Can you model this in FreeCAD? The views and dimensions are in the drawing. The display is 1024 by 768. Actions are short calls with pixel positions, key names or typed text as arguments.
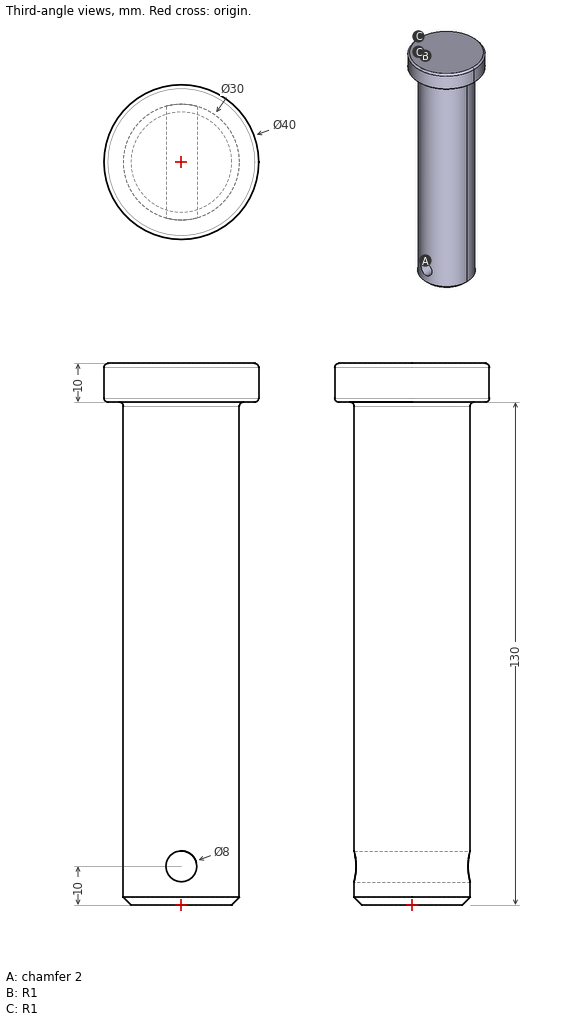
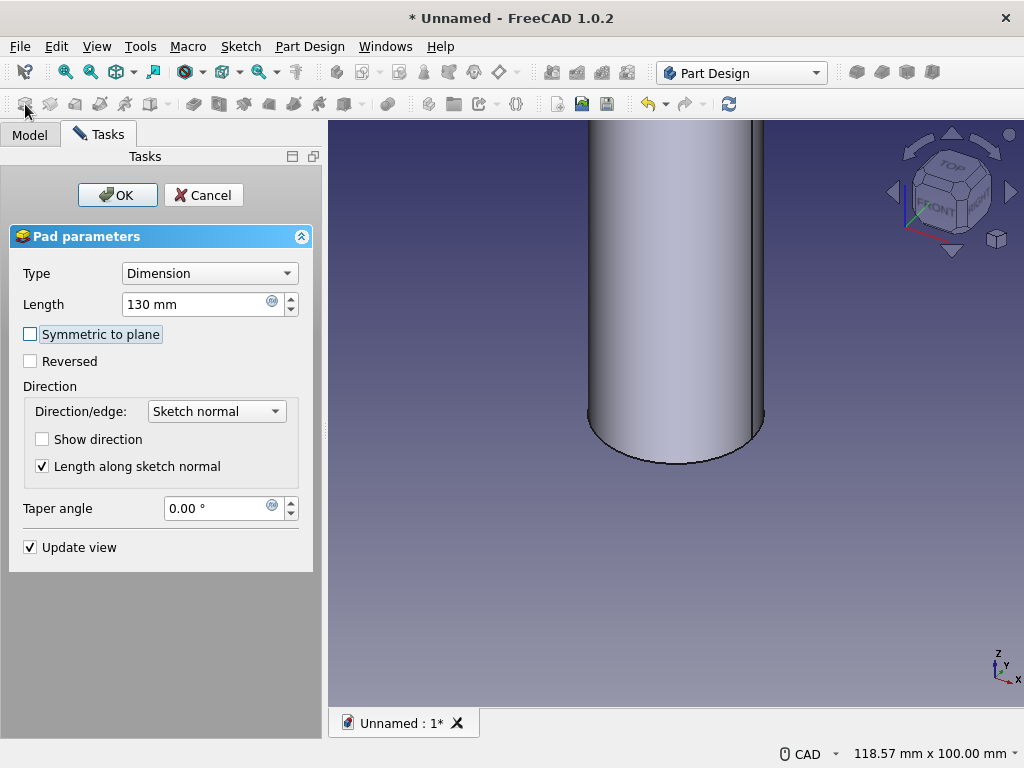
click(118, 195)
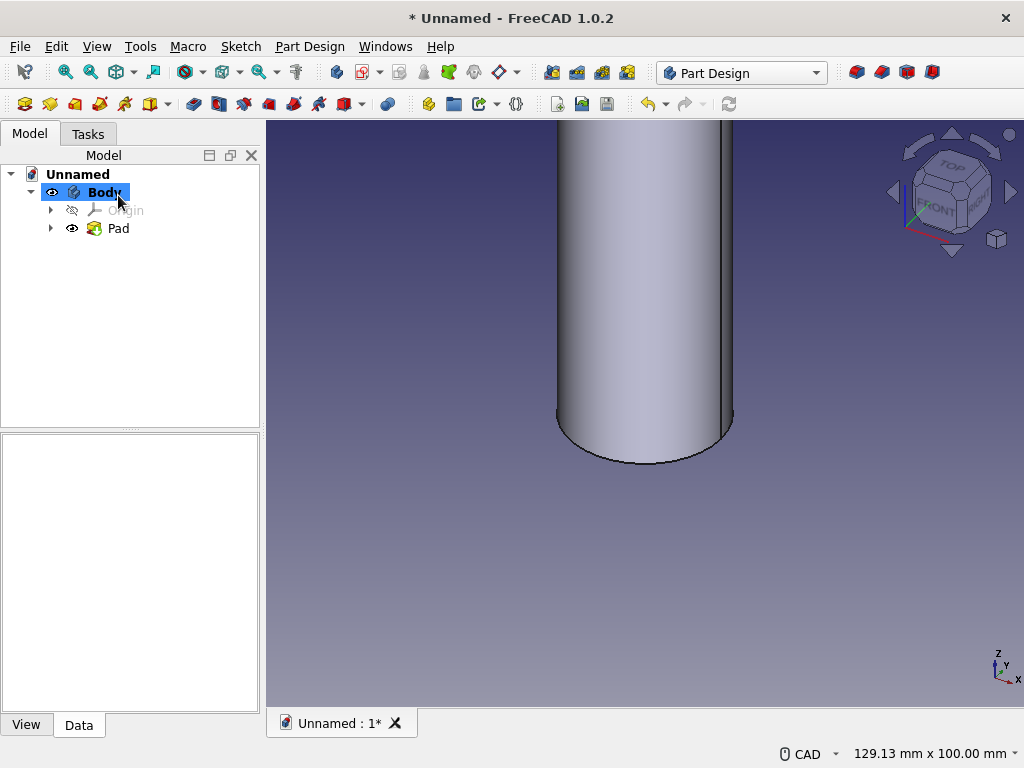
click(66, 72)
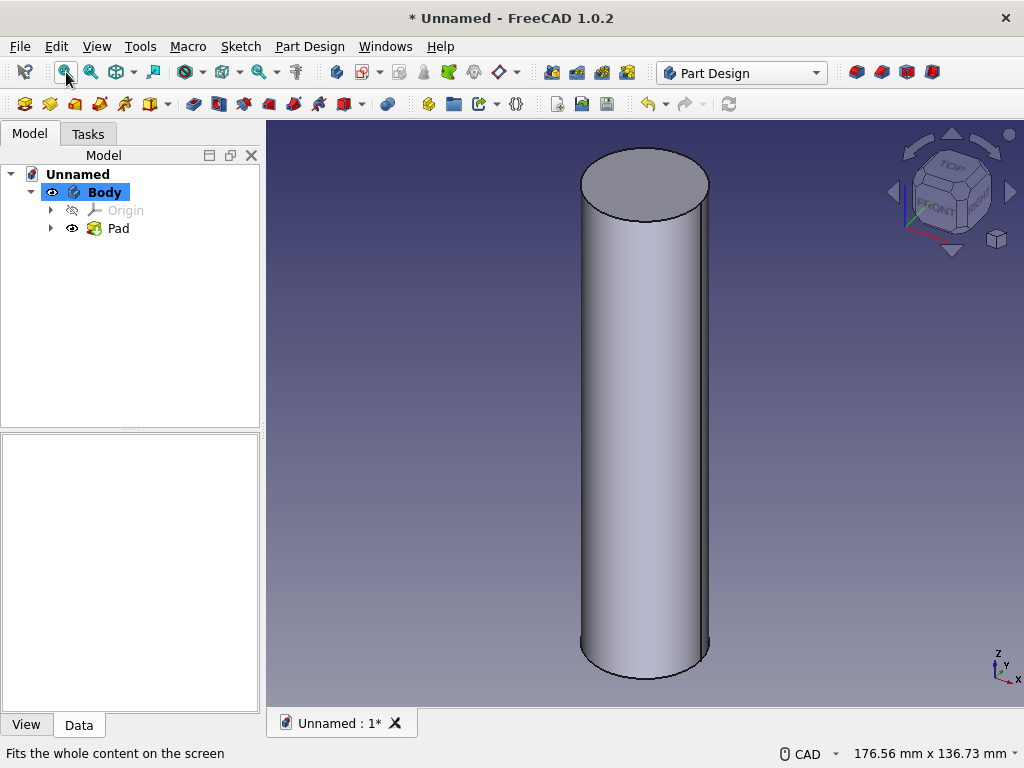
click(645, 184)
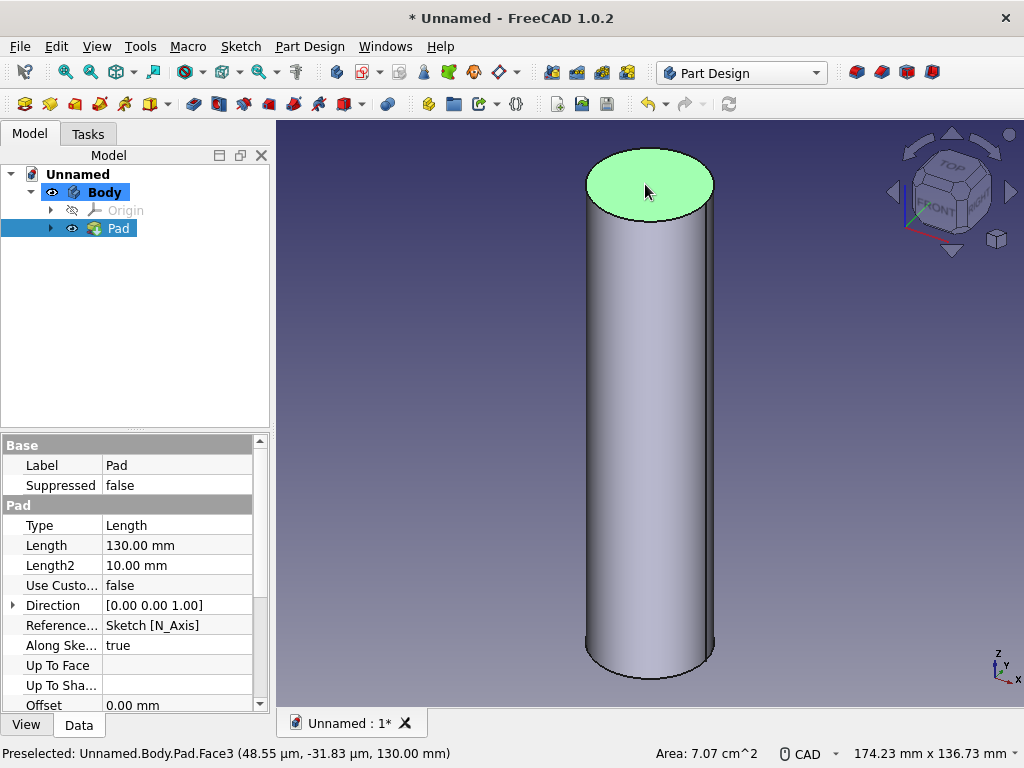
click(362, 72)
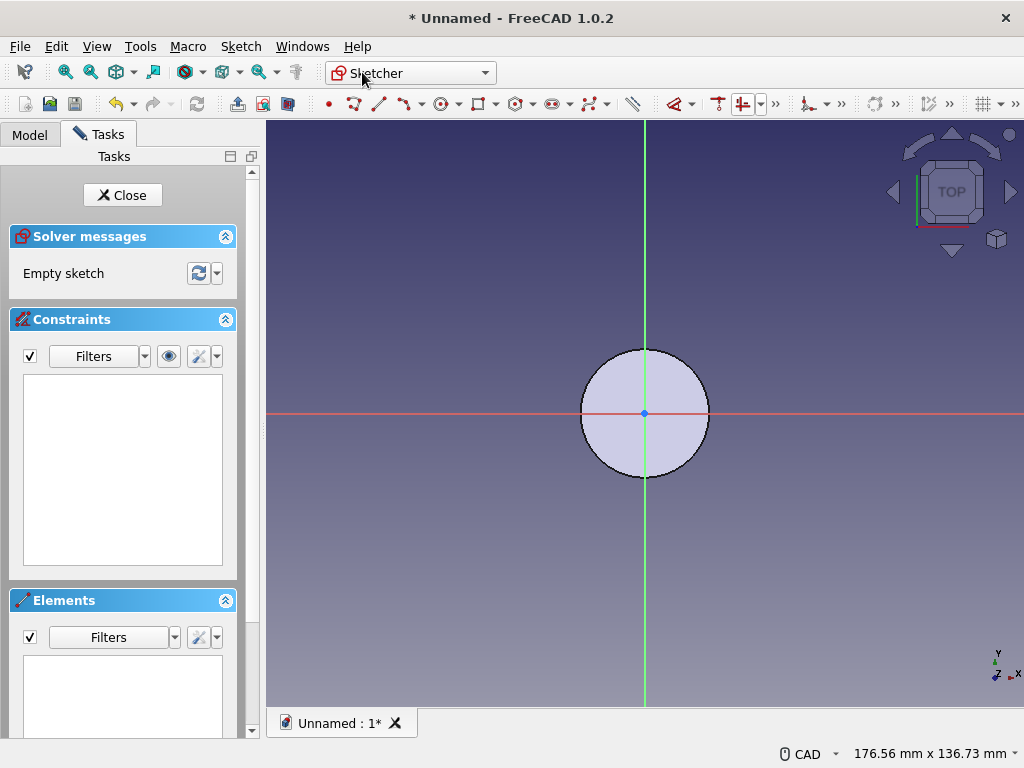
scroll(701, 413, up, 4)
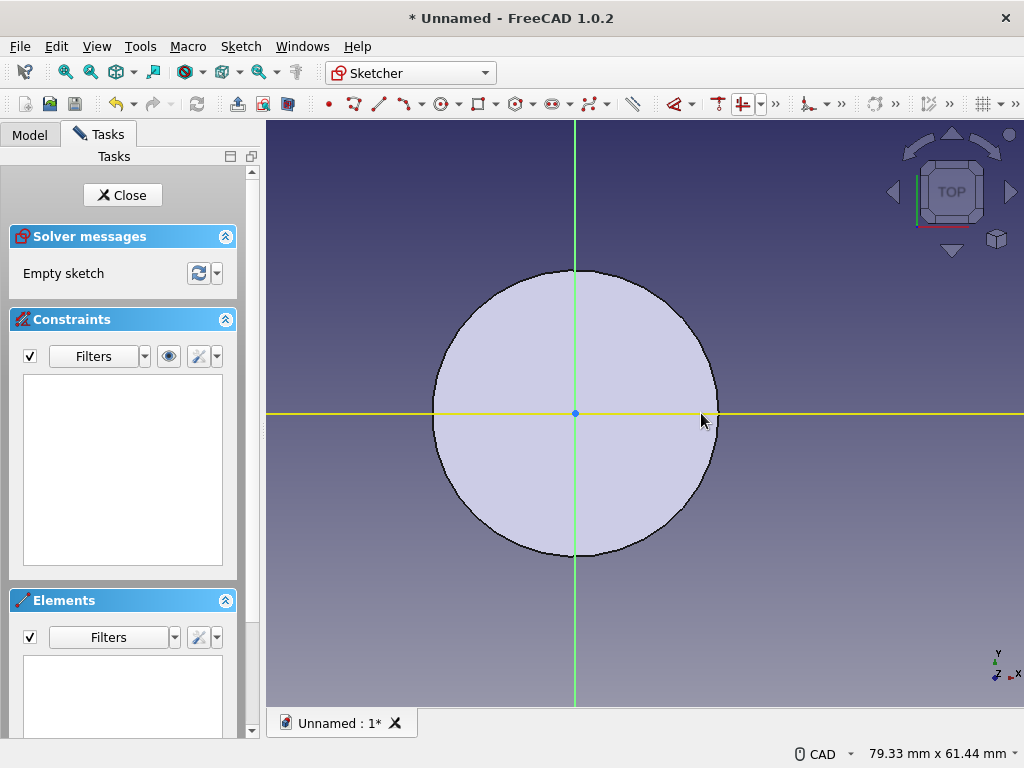
click(440, 104)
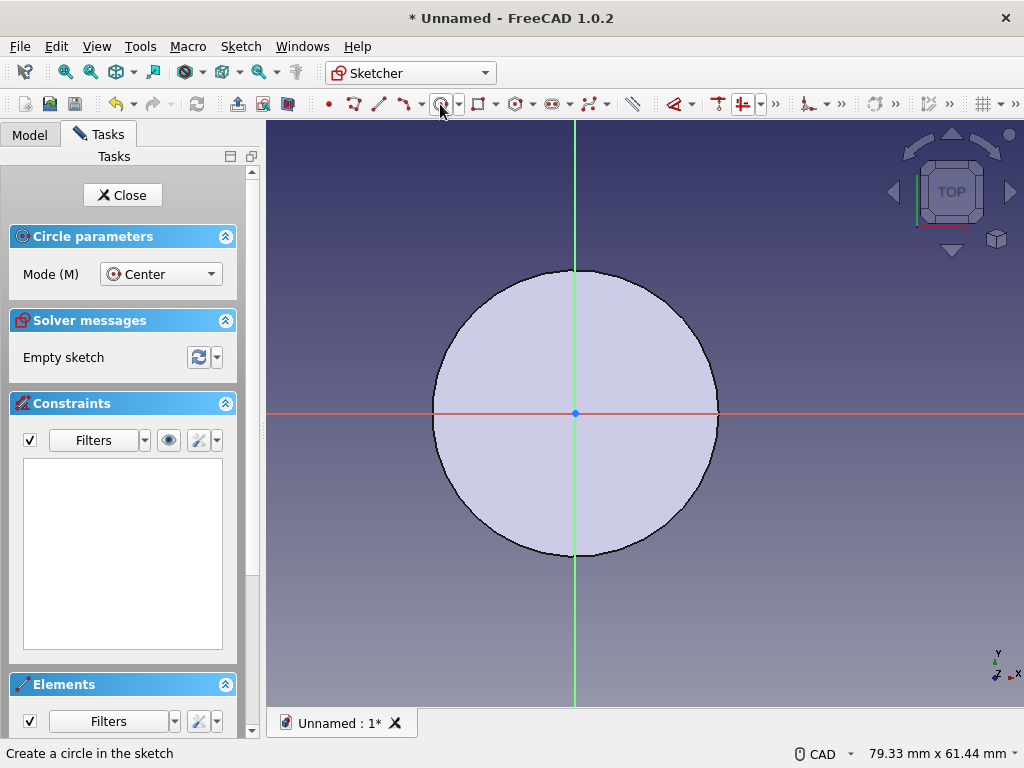
click(575, 414)
click(711, 278)
key(Escape)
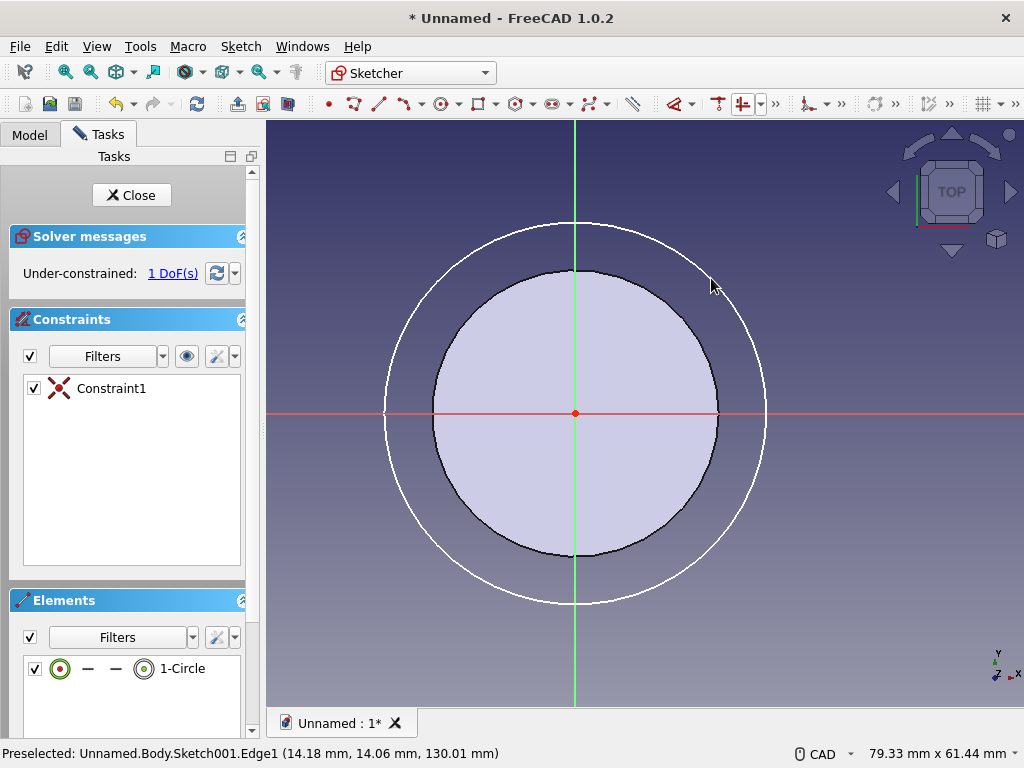
click(674, 104)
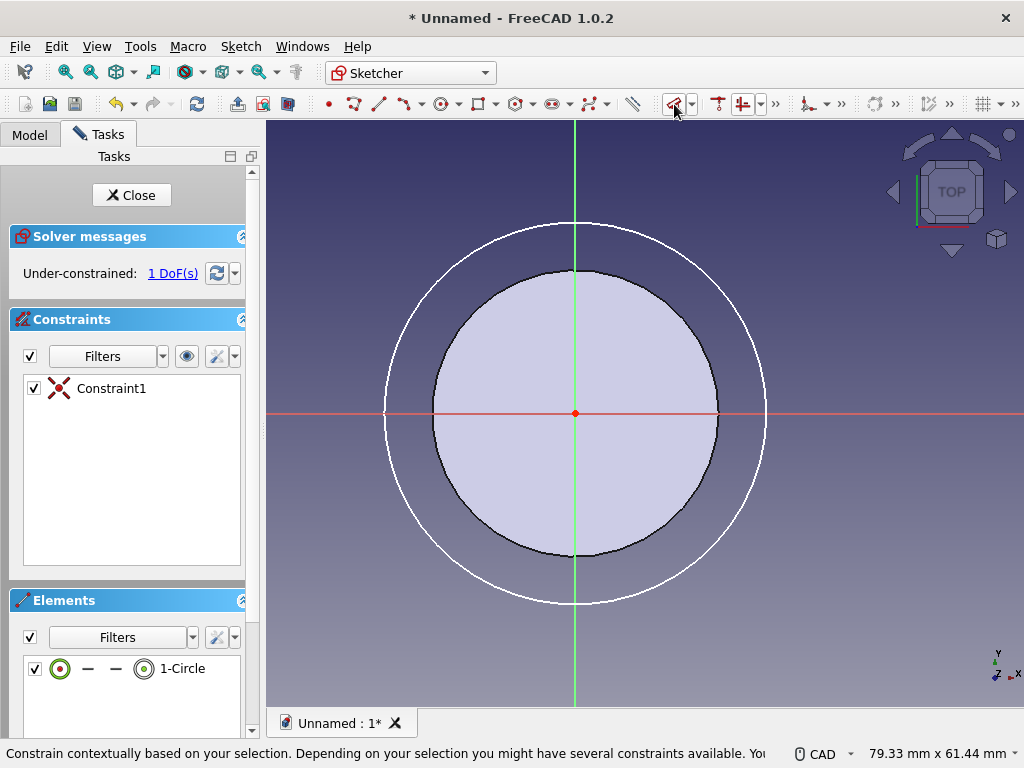
click(710, 278)
click(733, 255)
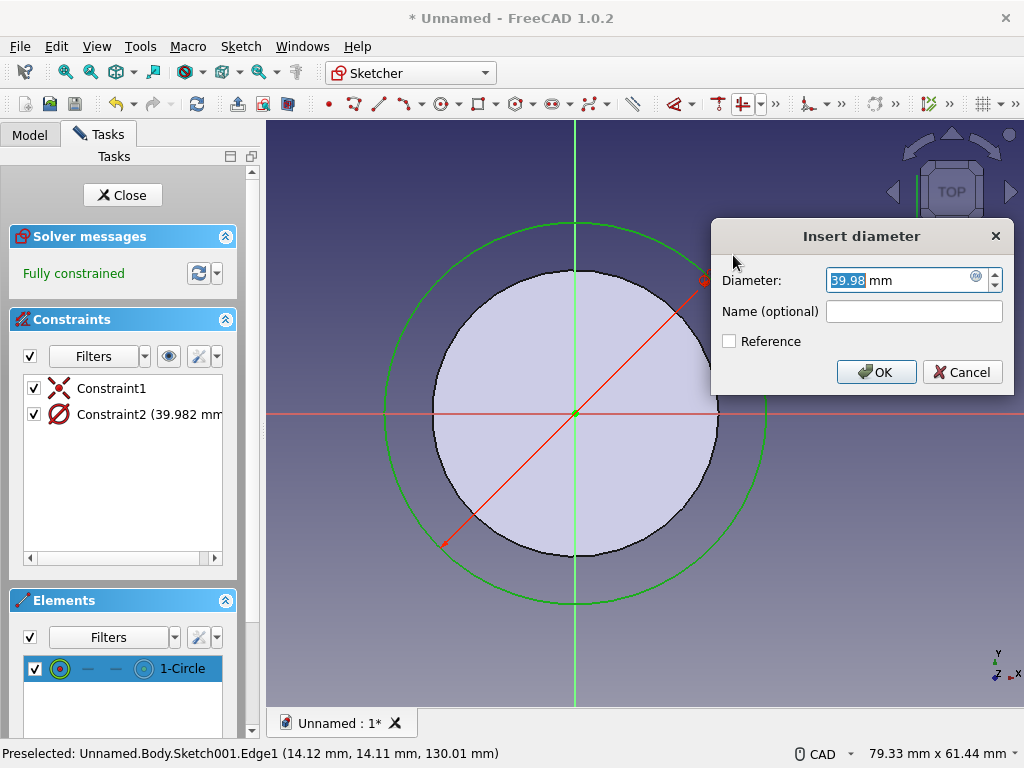
text(40)
key(Return)
key(Escape)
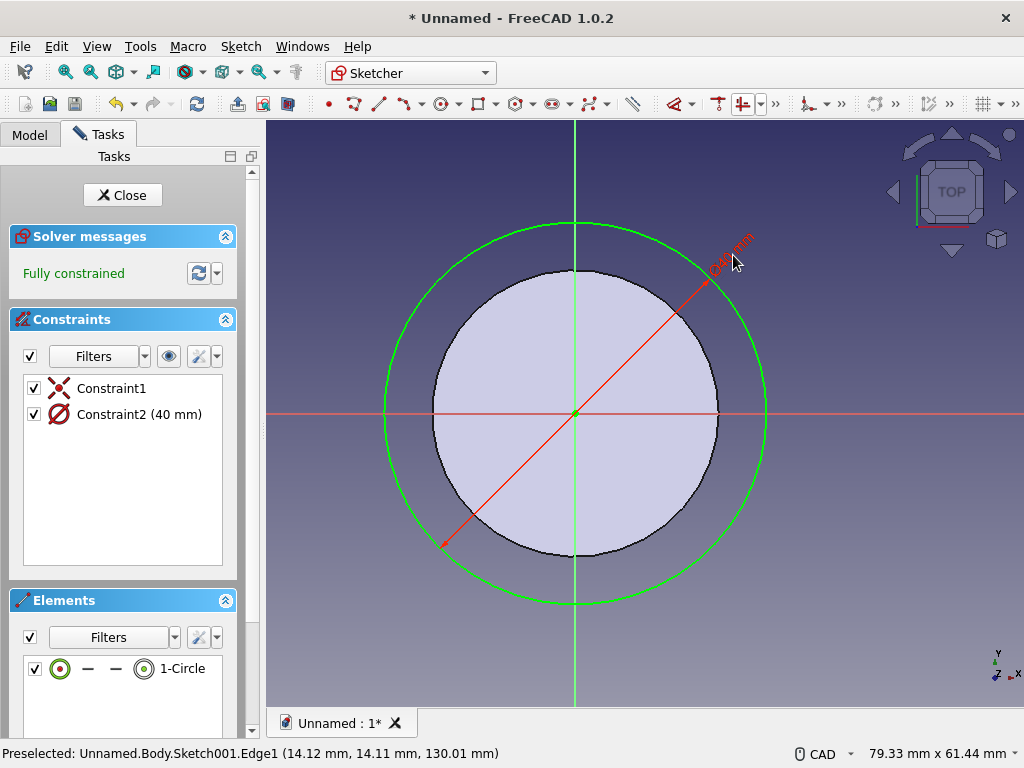
click(123, 195)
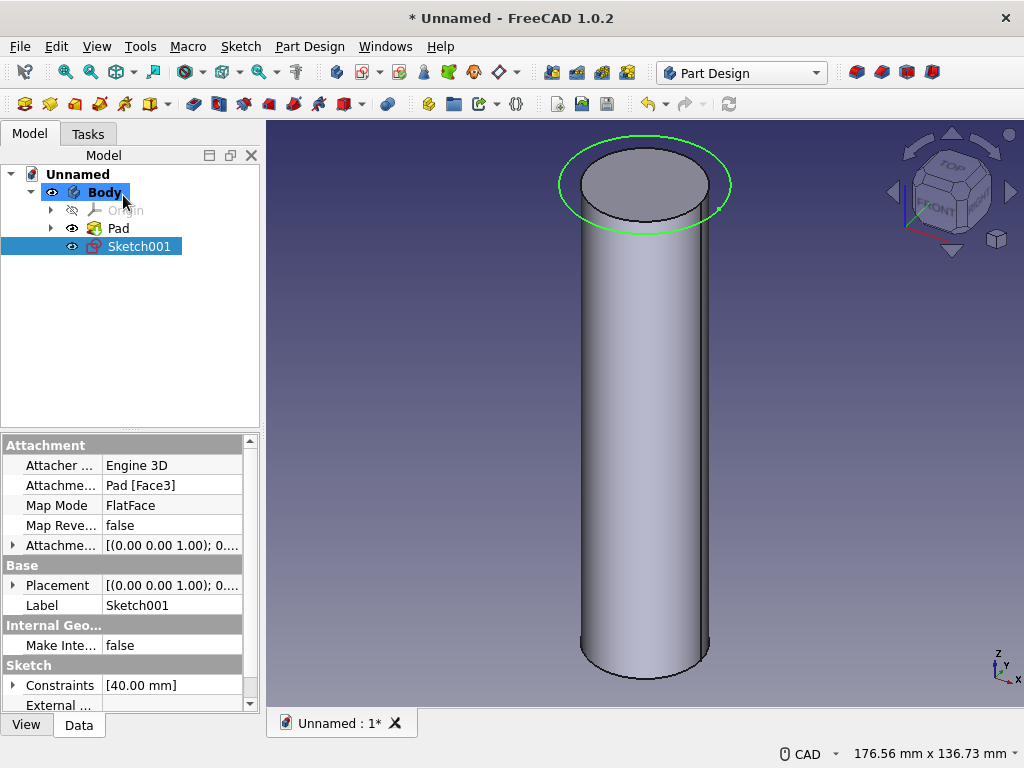
click(25, 104)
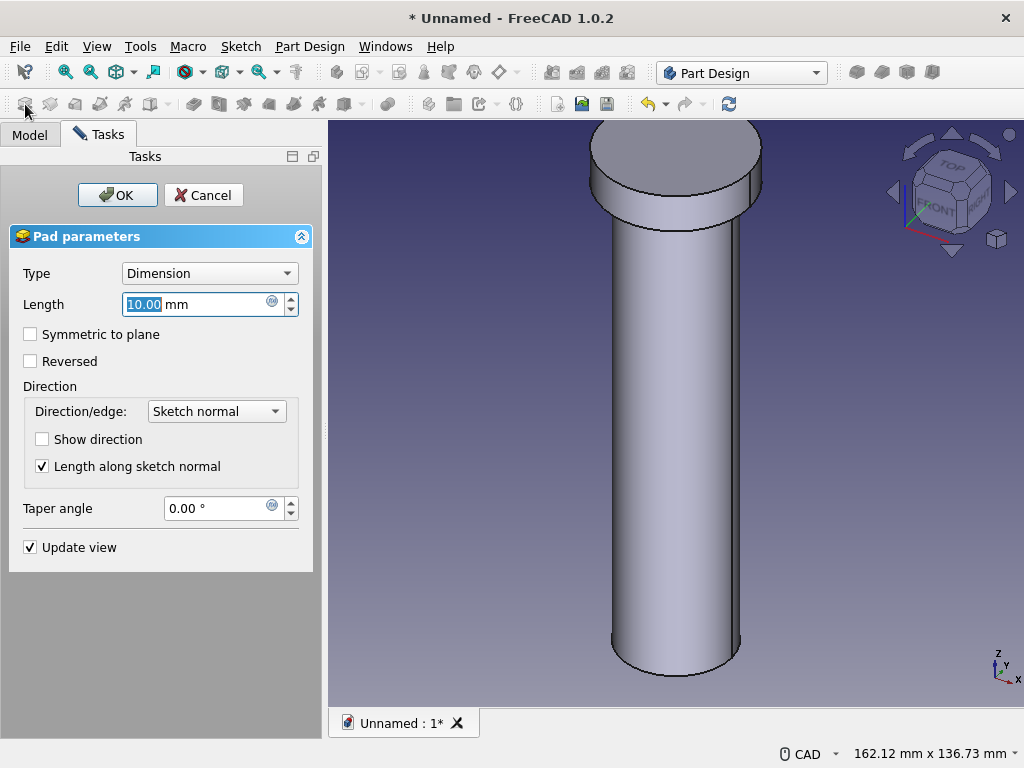
text(10)
key(Tab)